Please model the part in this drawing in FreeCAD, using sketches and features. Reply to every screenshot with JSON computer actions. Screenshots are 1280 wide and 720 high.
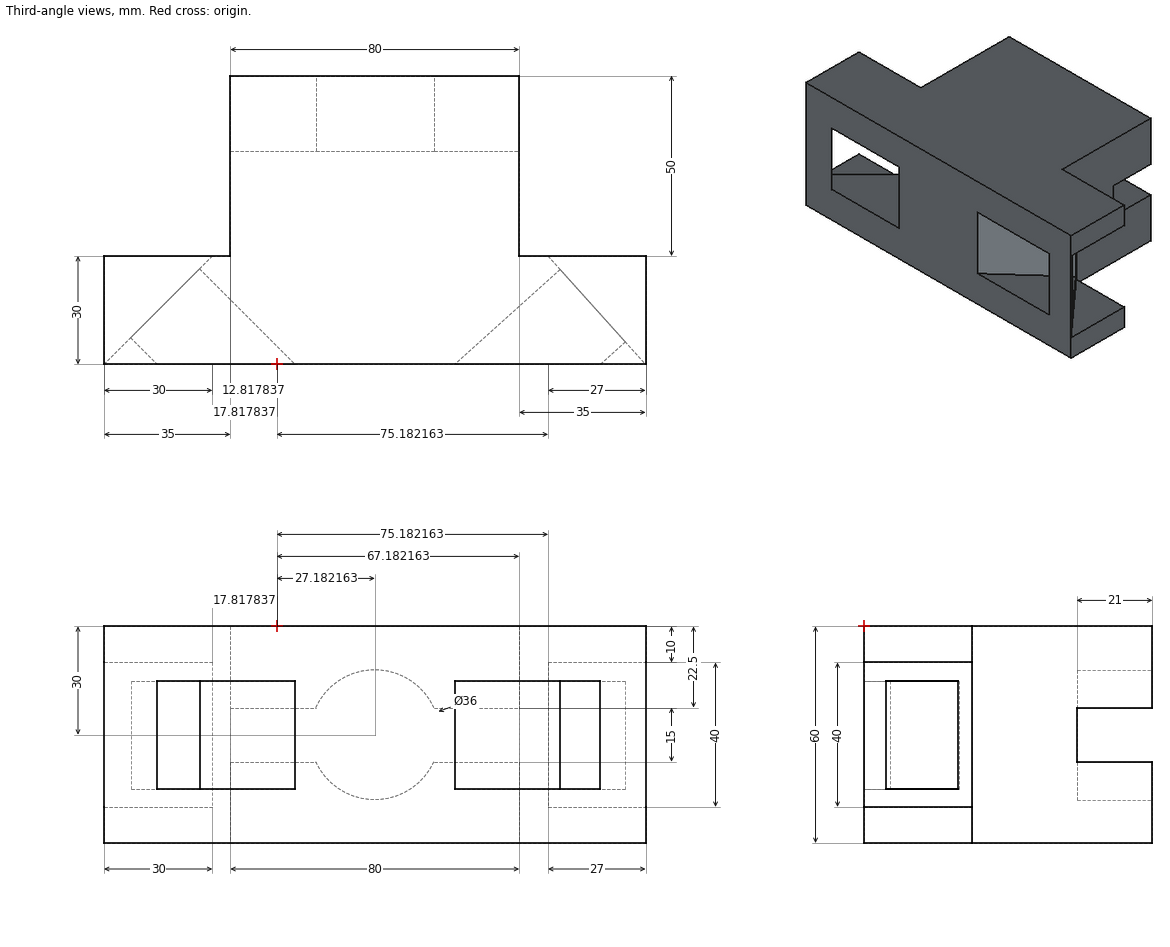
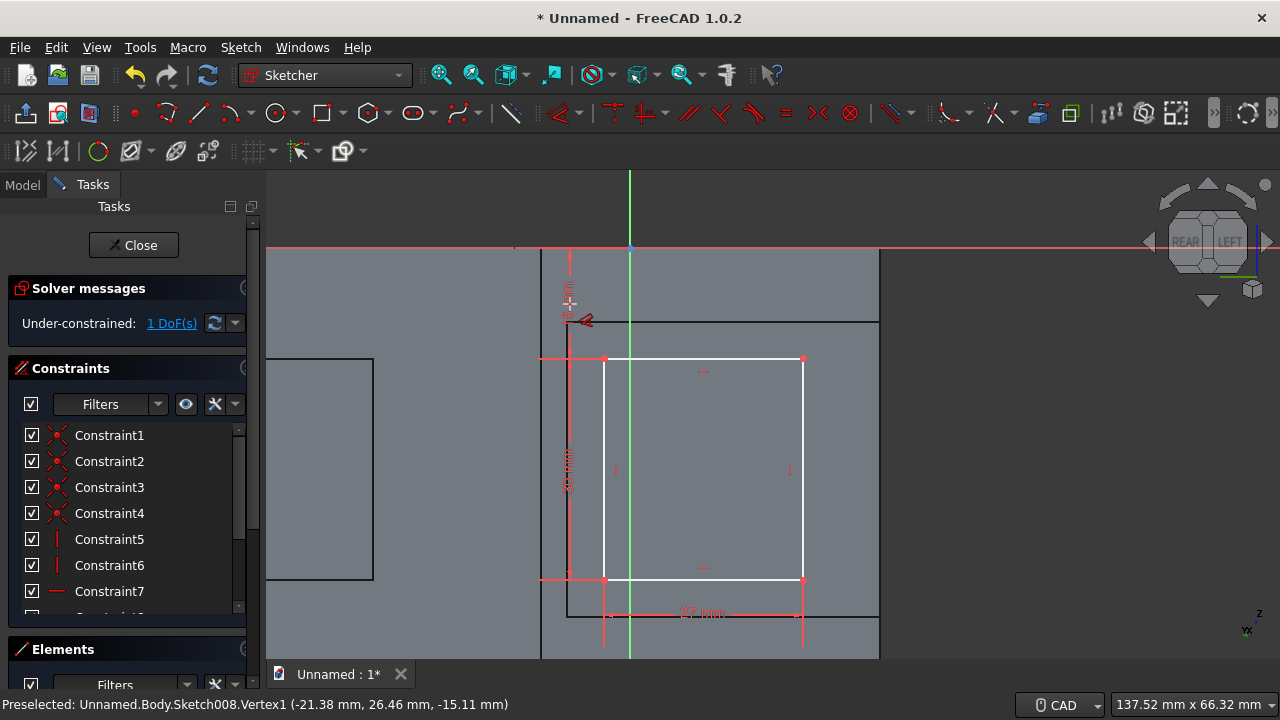
{"action": "scroll", "coordinate": [604, 359], "scroll_direction": "up", "scroll_amount": 2}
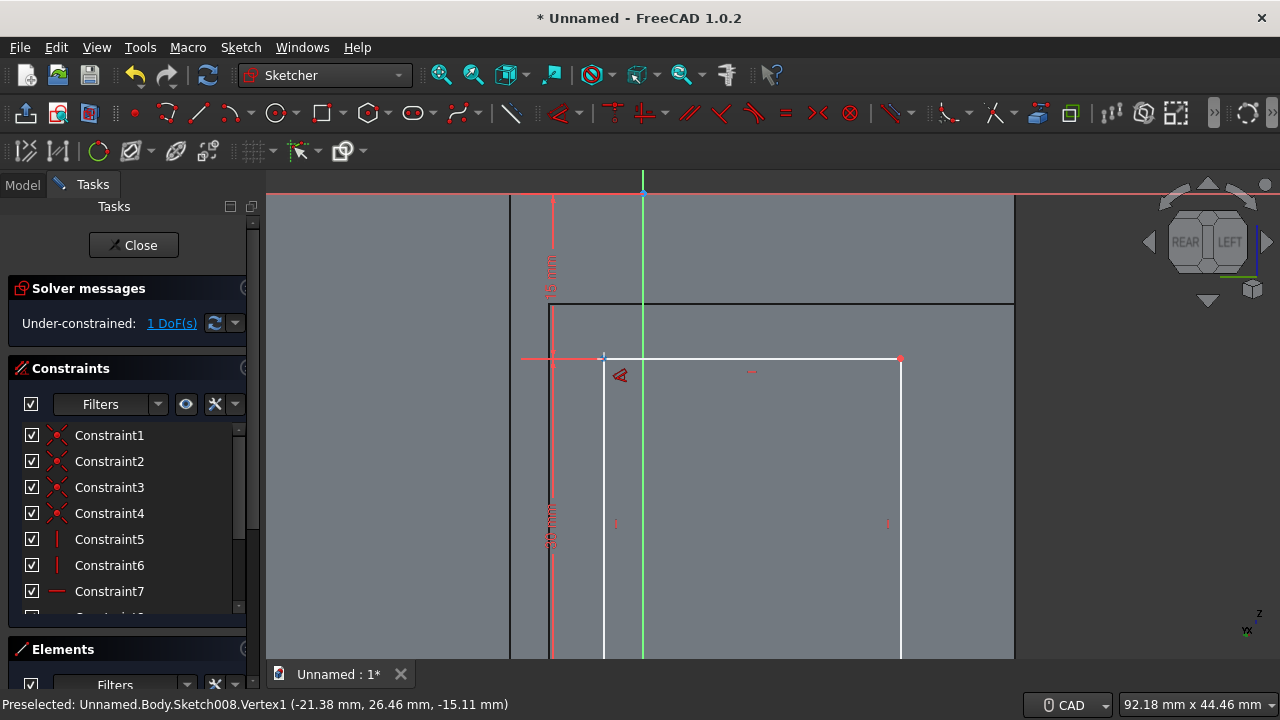
{"action": "left_click", "coordinate": [604, 359]}
{"action": "left_click", "coordinate": [624, 393]}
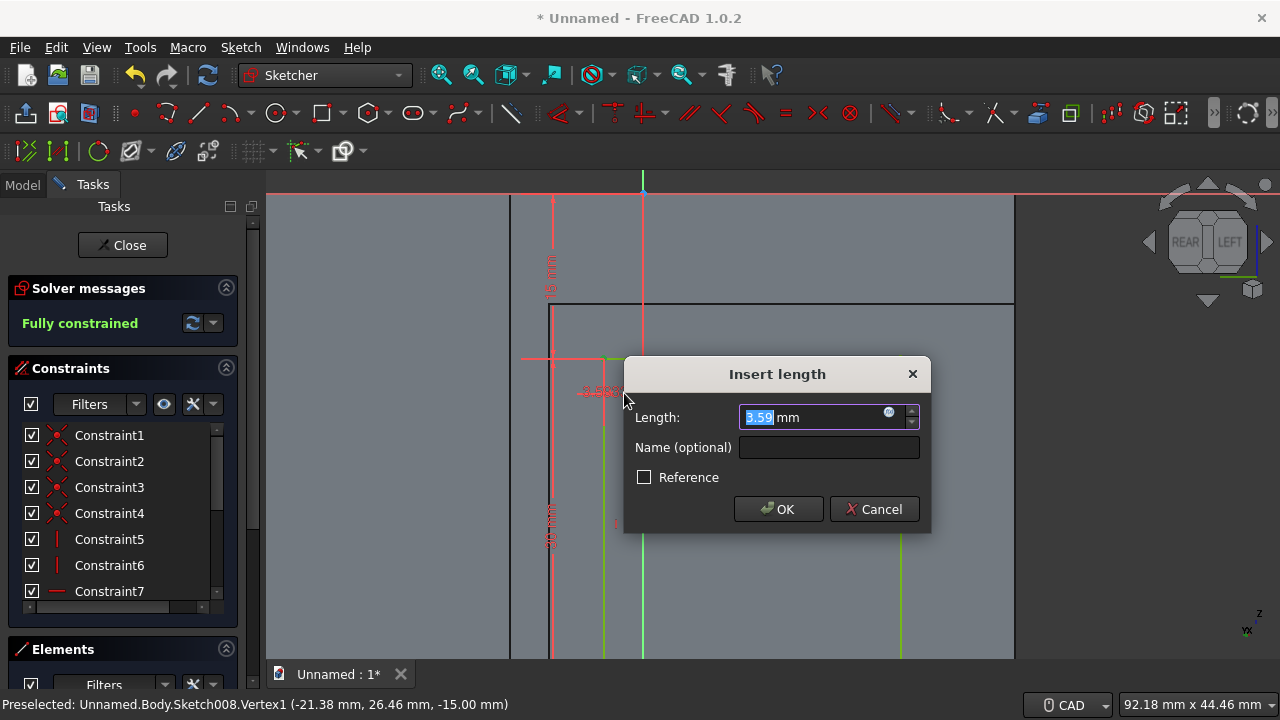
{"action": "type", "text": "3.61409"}
{"action": "key", "text": "Return"}
{"action": "key", "text": "Escape"}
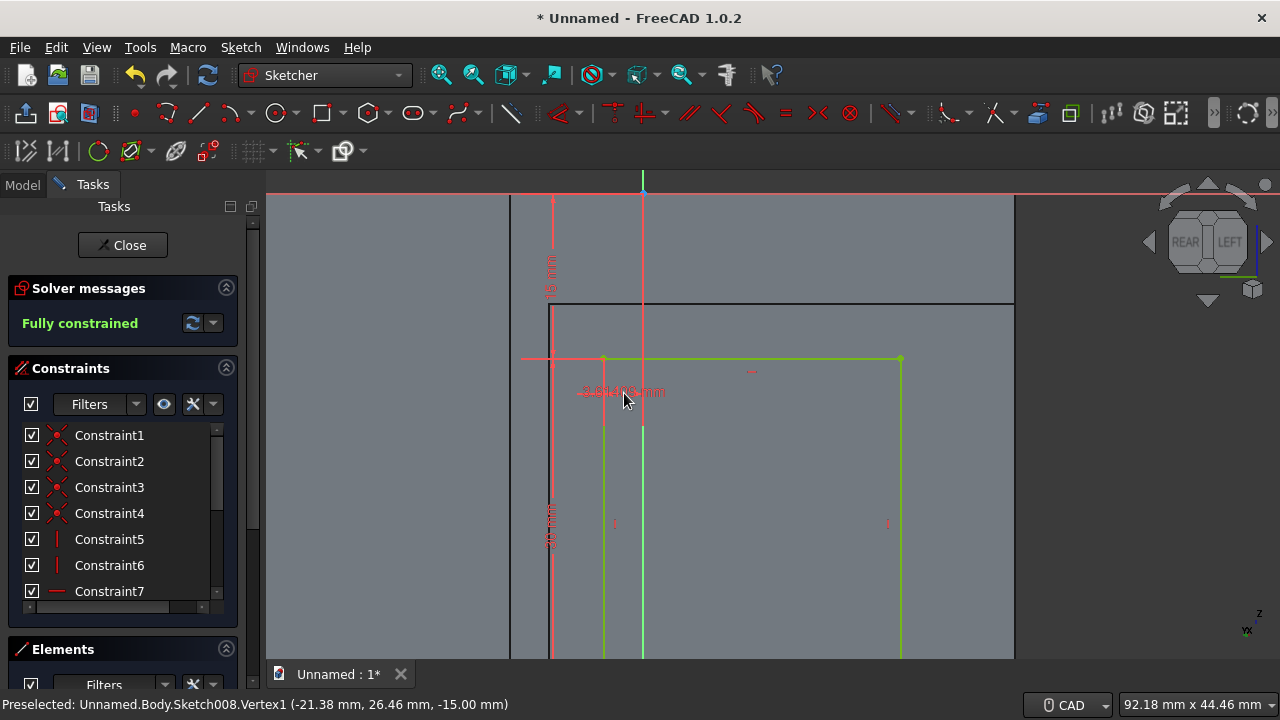
{"action": "left_click", "coordinate": [123, 245]}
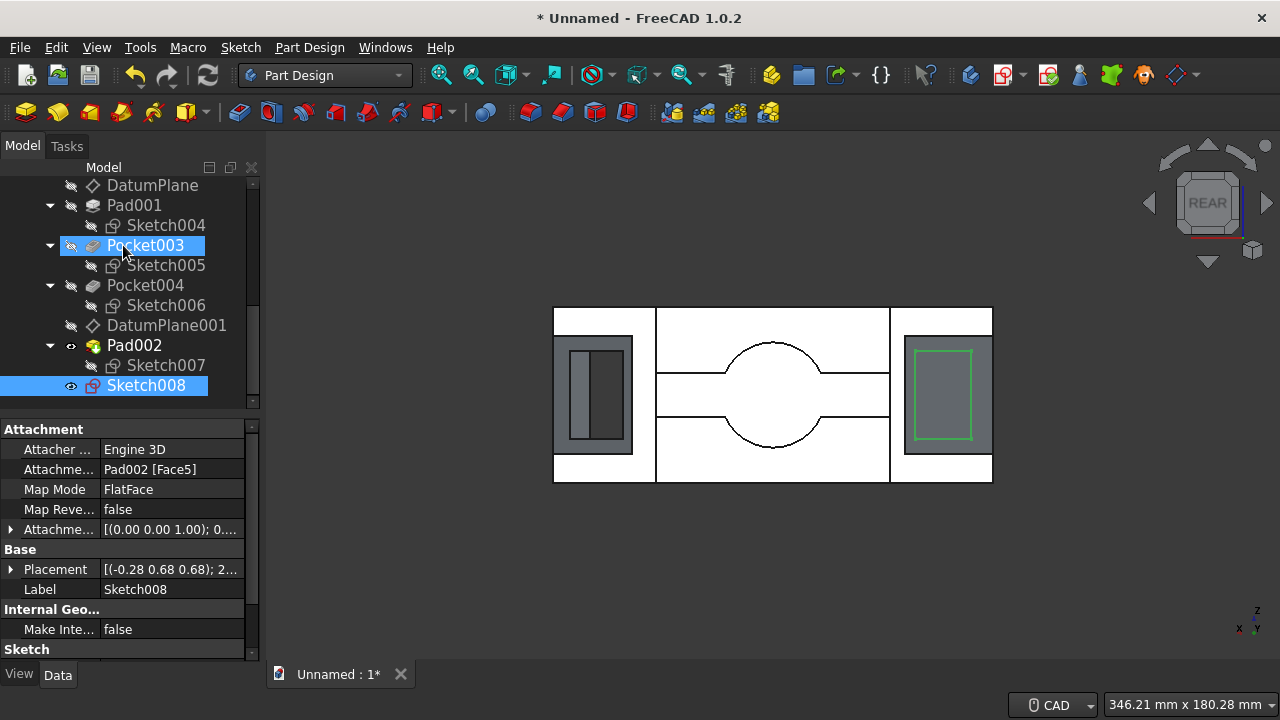
{"action": "left_click", "coordinate": [240, 112]}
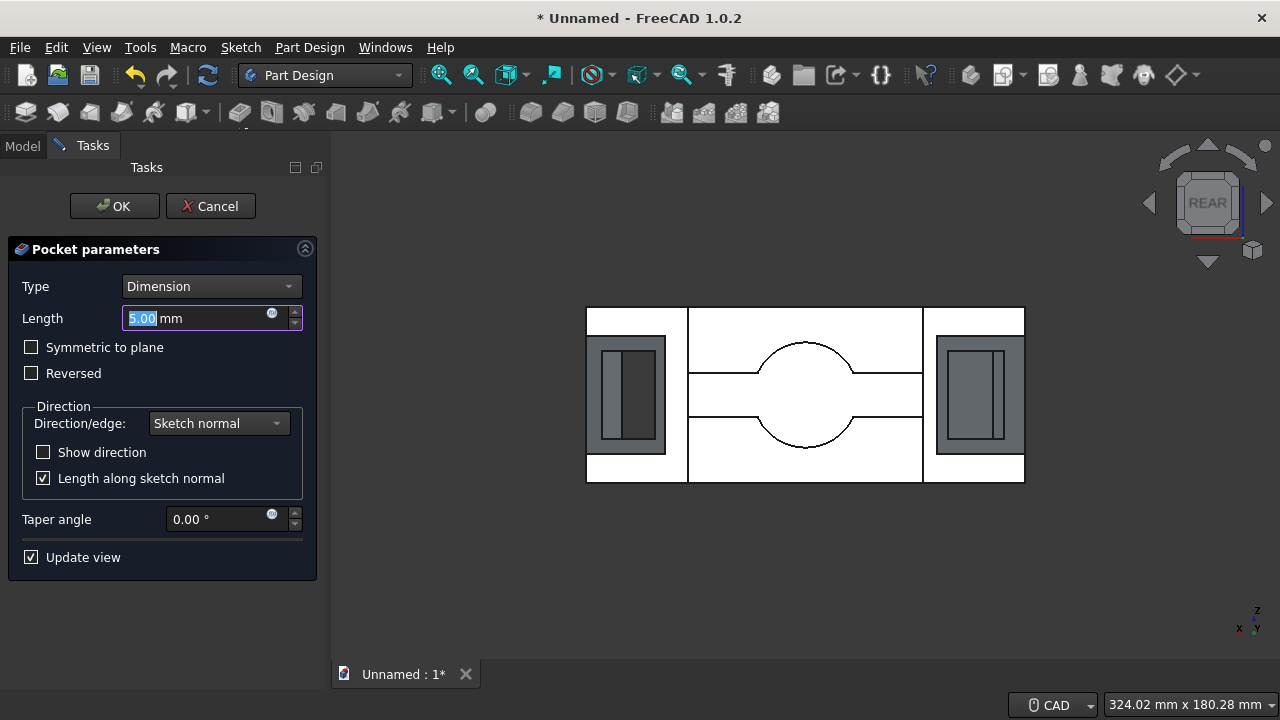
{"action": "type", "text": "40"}
{"action": "key", "text": "Tab"}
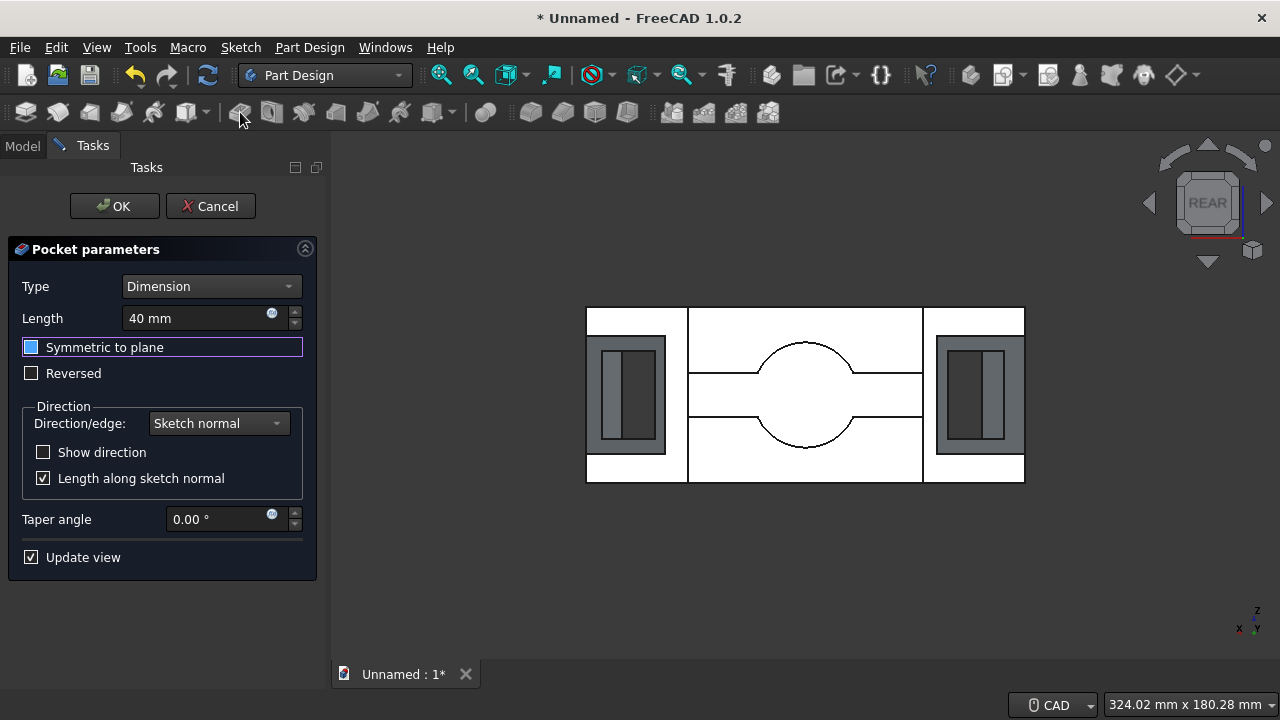
{"action": "left_click", "coordinate": [115, 206]}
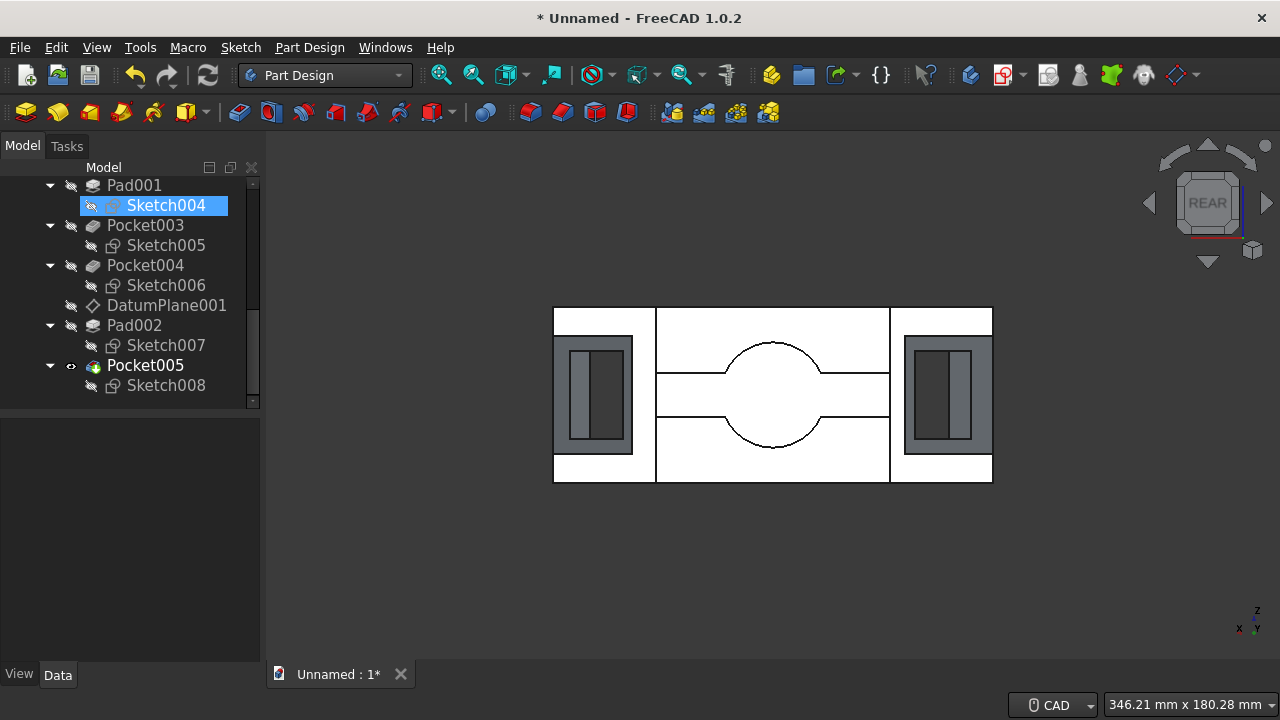
{"action": "key", "text": "0"}